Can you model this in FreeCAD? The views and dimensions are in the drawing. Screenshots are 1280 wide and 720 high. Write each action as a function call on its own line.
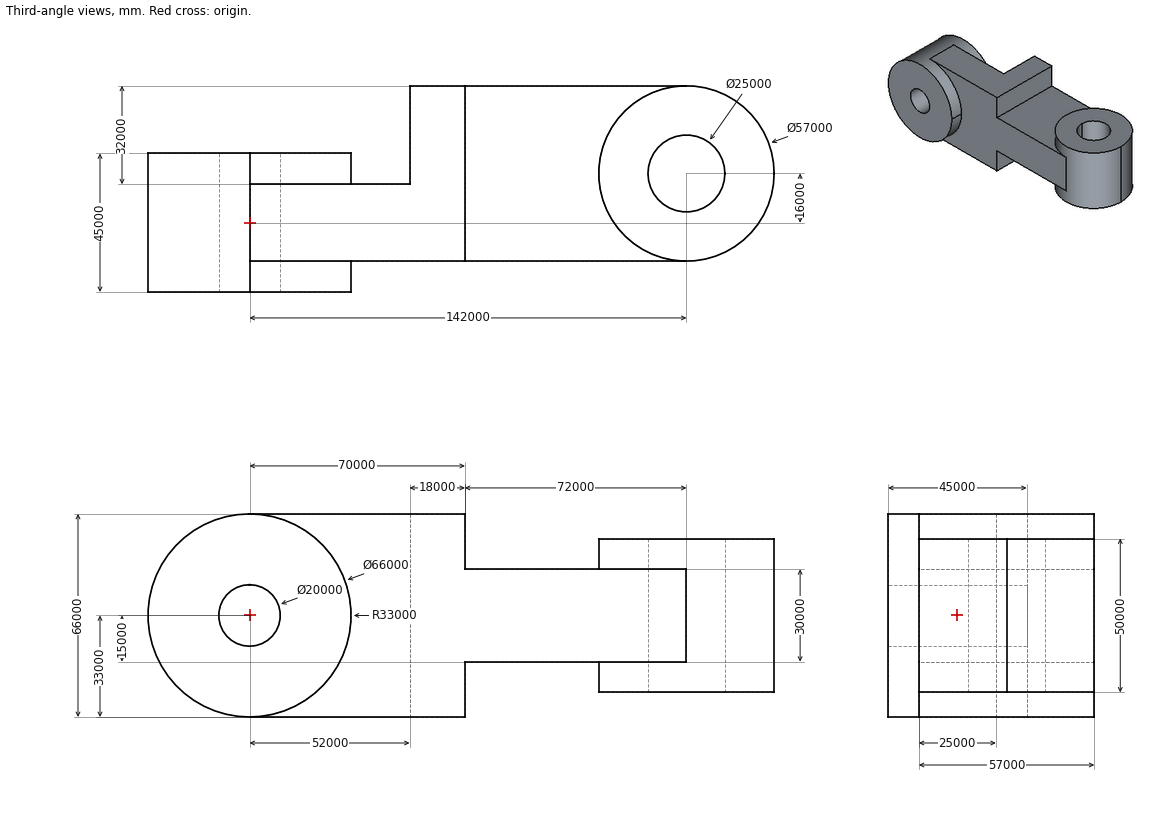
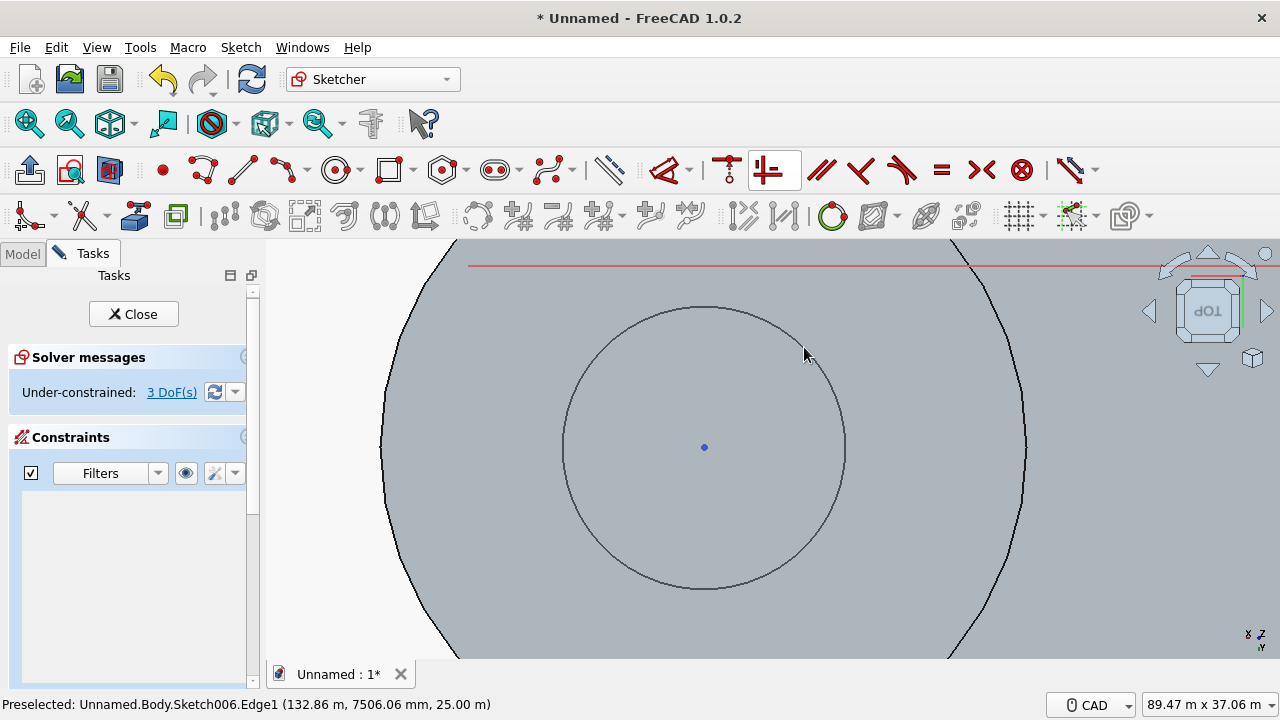
click(664, 170)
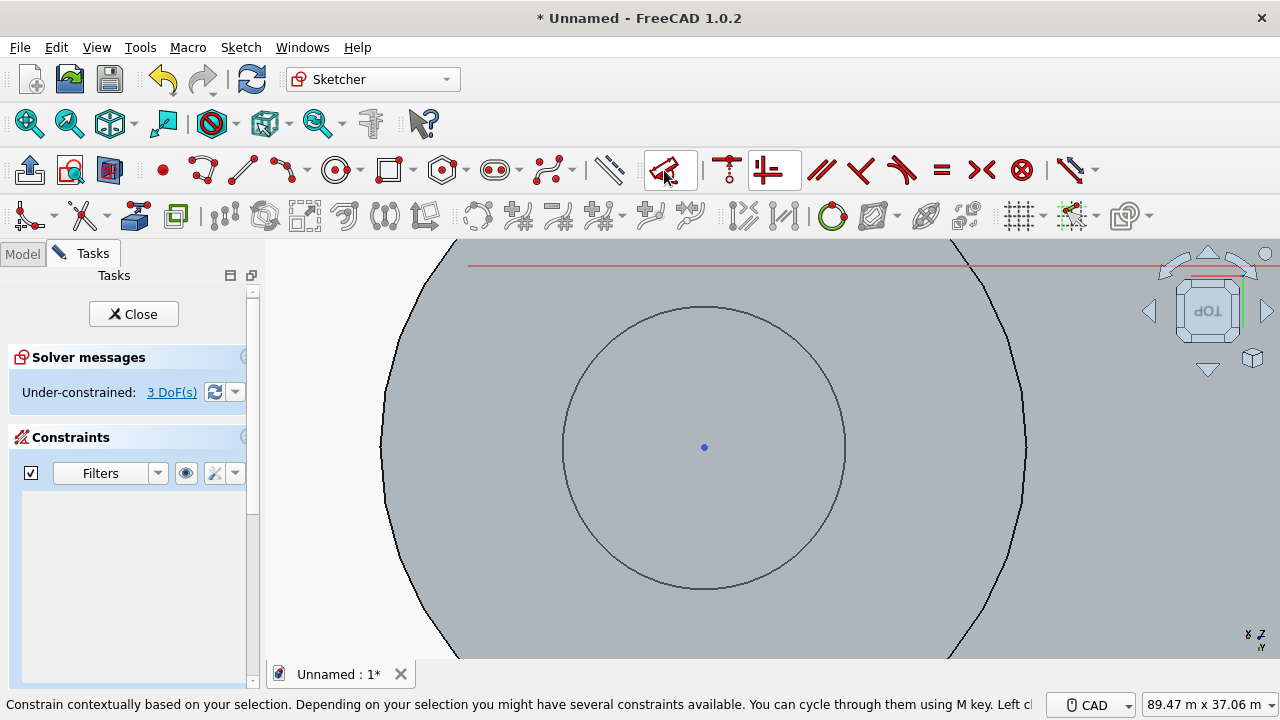
click(804, 348)
click(827, 325)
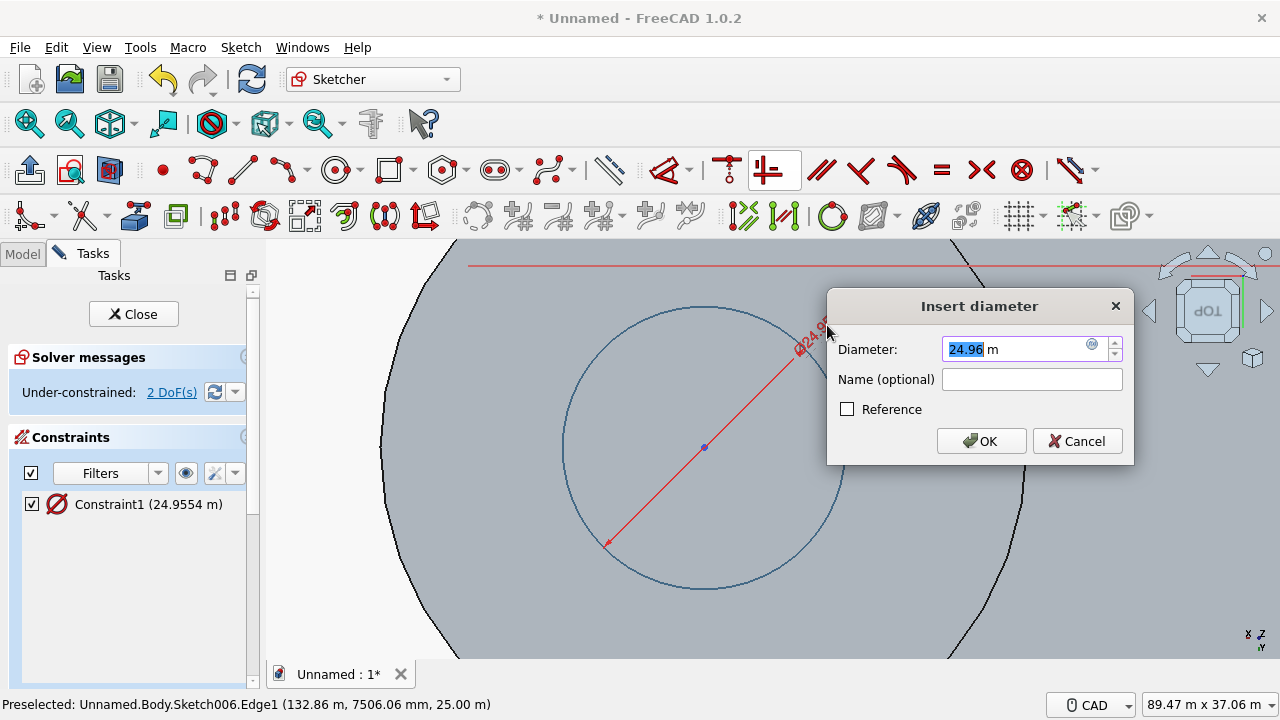
key(ctrl+a)
text(25000 mm)
key(Return)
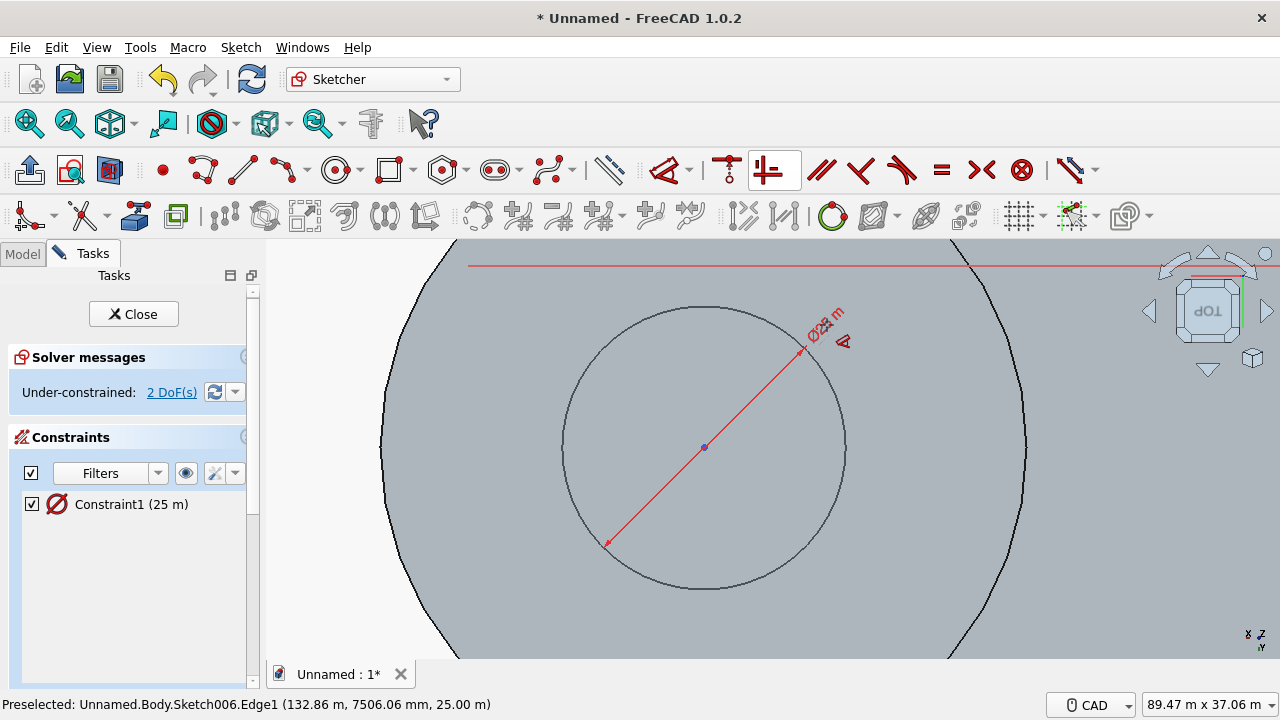
click(704, 448)
click(670, 357)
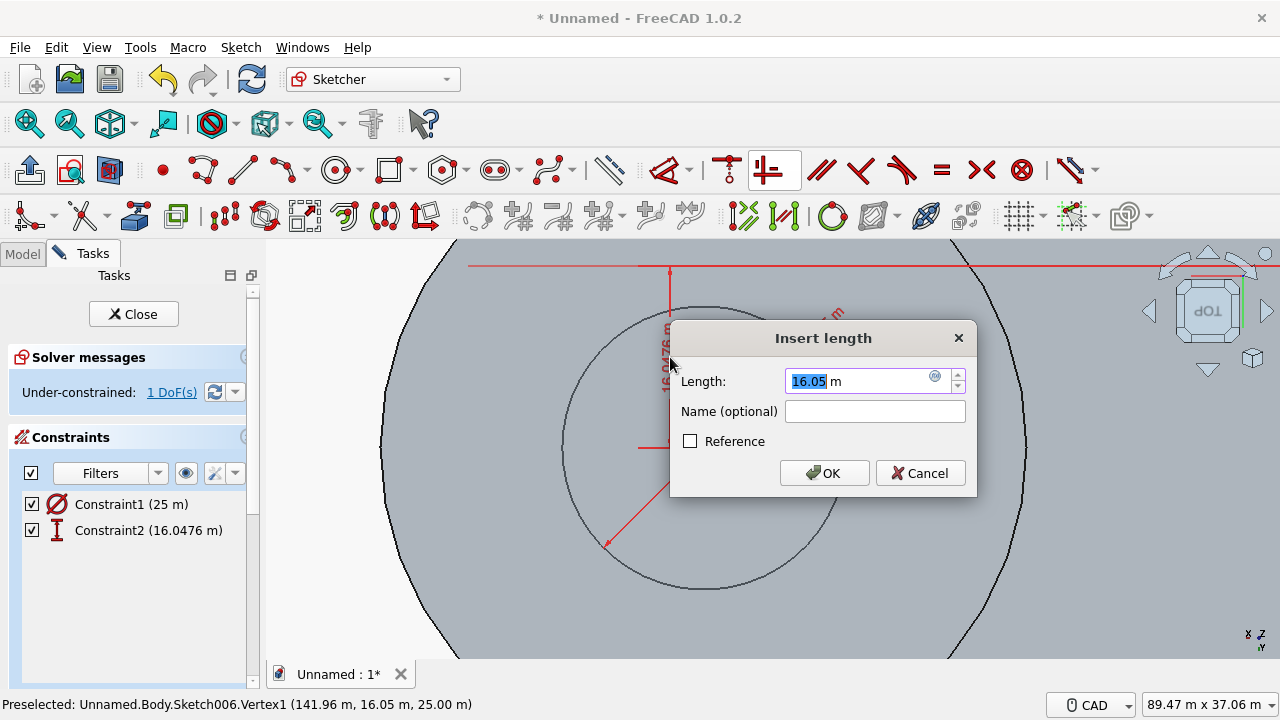
key(ctrl+a)
text(16000 mm)
key(Return)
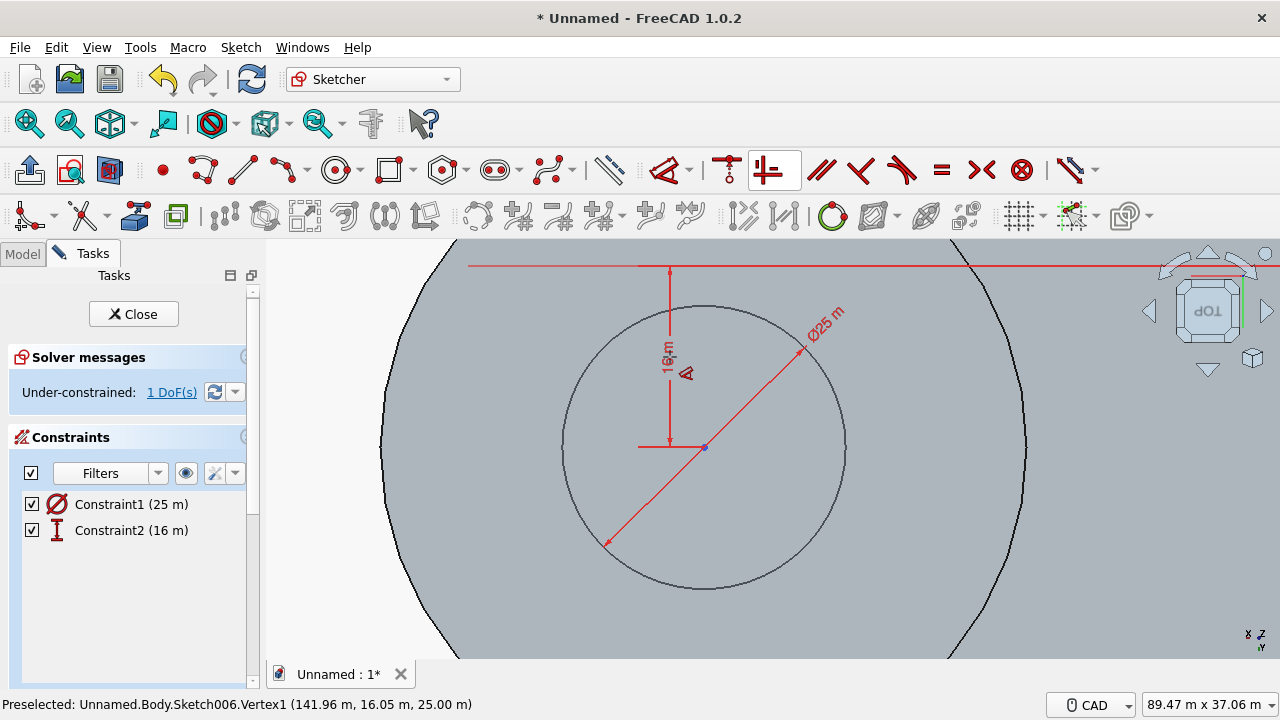
click(704, 447)
click(910, 481)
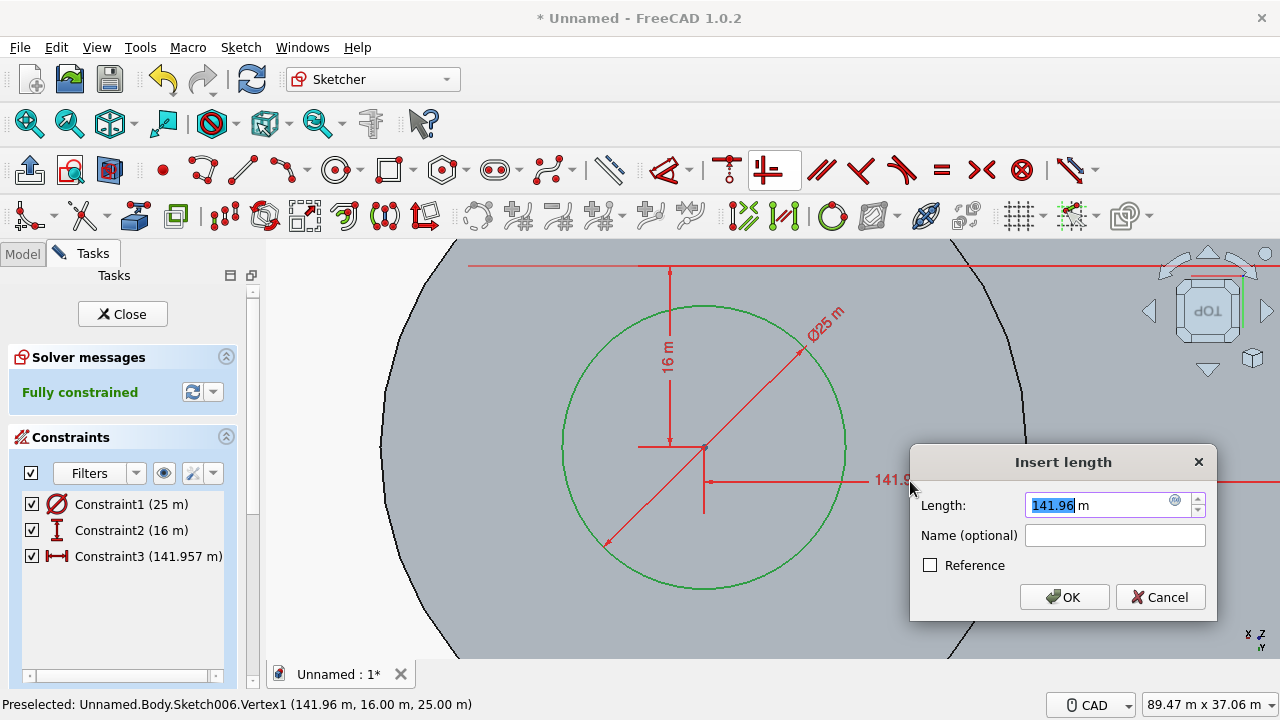
key(ctrl+a)
text(142000 mm)
key(Return)
key(Escape)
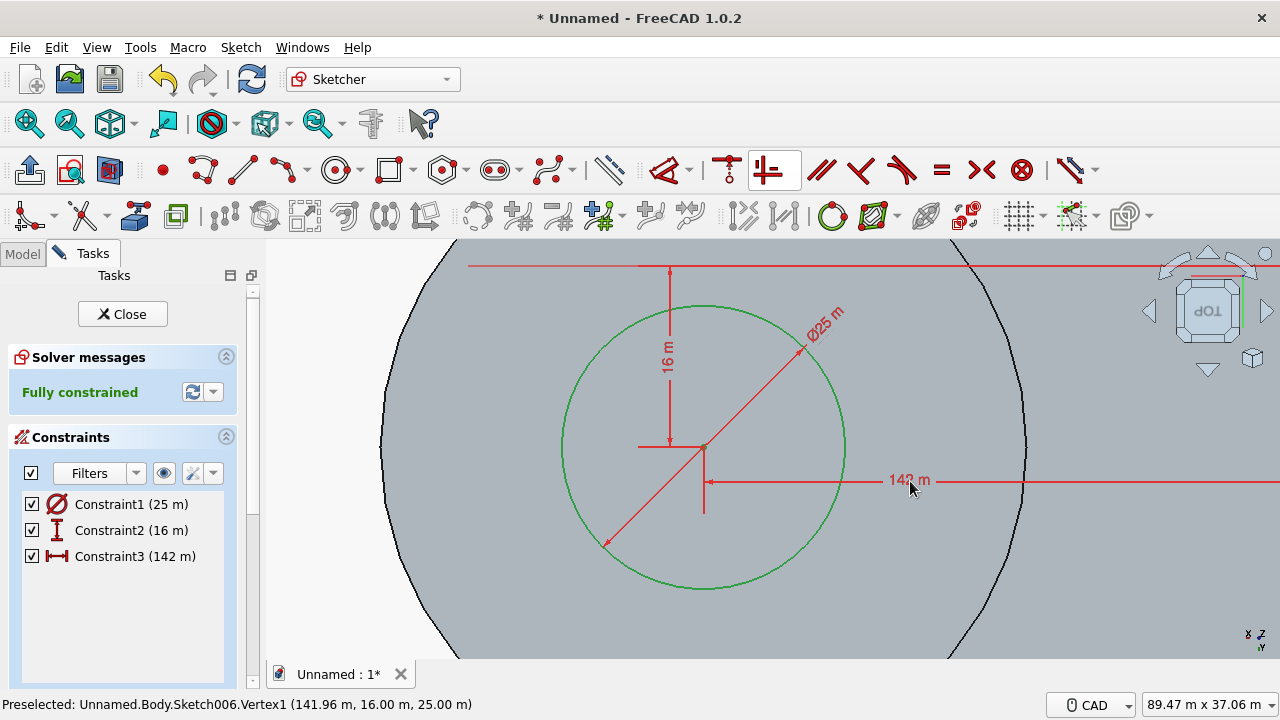
click(123, 314)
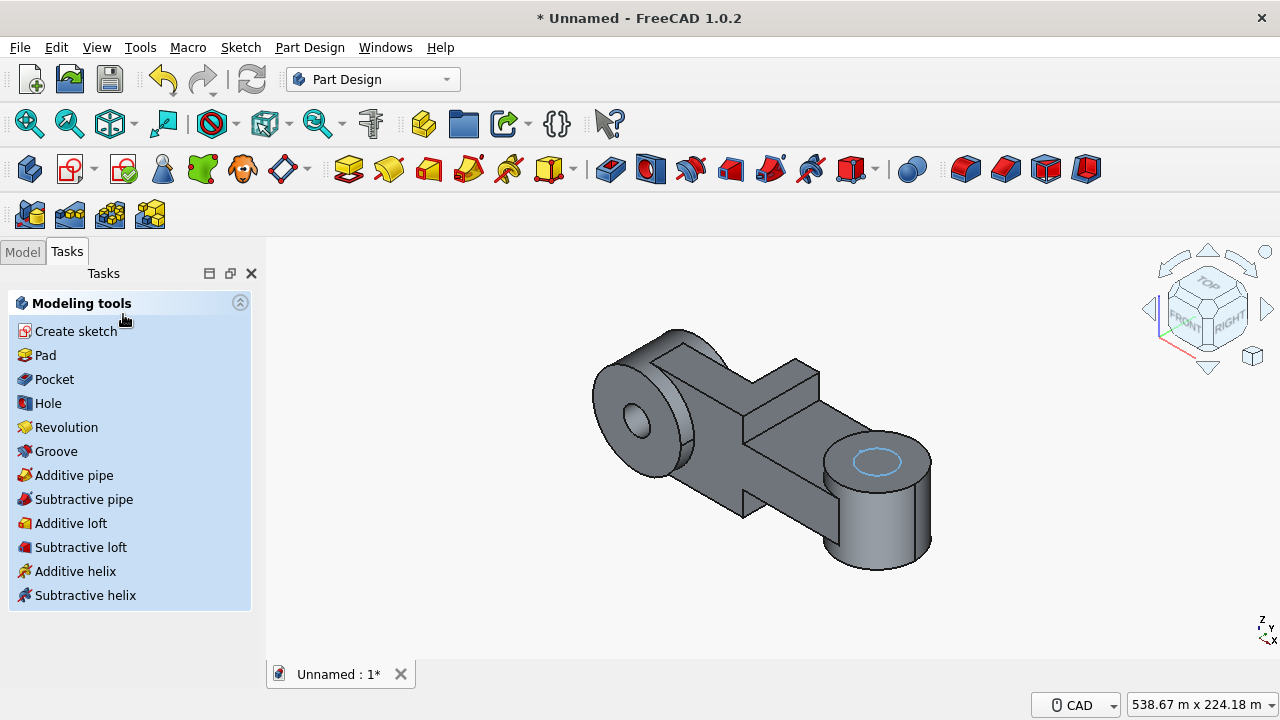
click(612, 170)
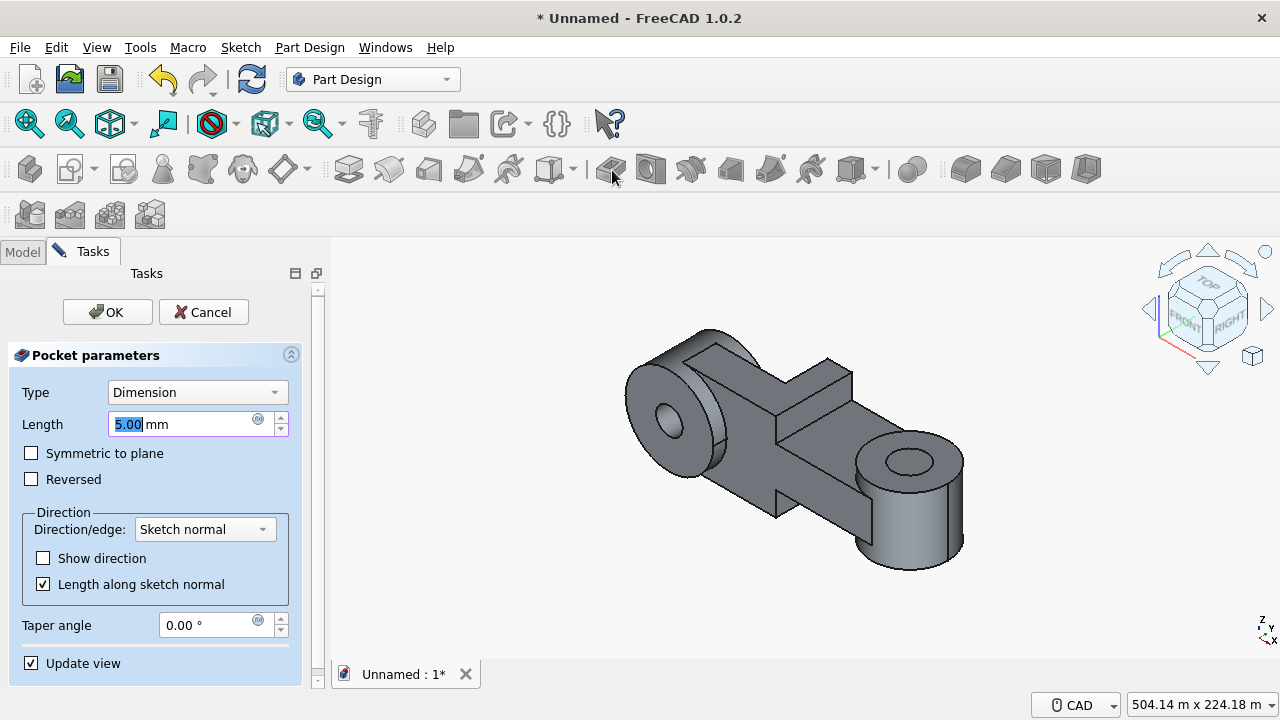
text(50000)
key(Tab)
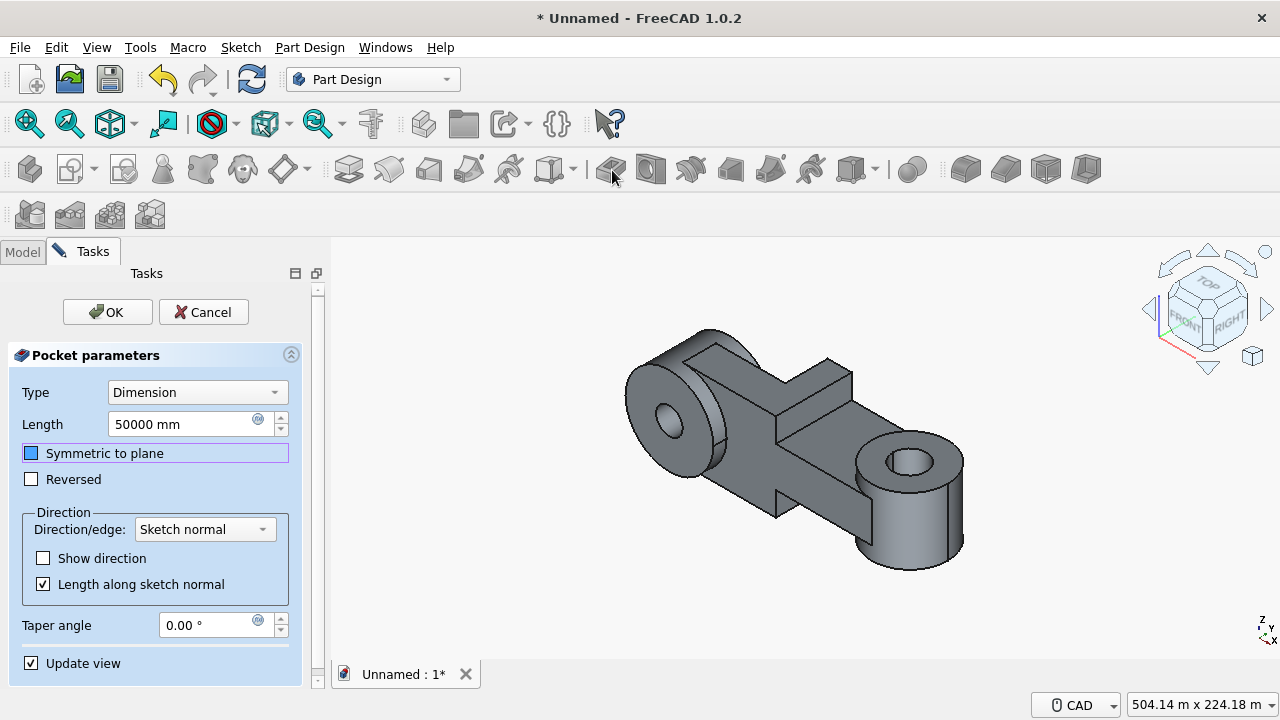
click(108, 312)